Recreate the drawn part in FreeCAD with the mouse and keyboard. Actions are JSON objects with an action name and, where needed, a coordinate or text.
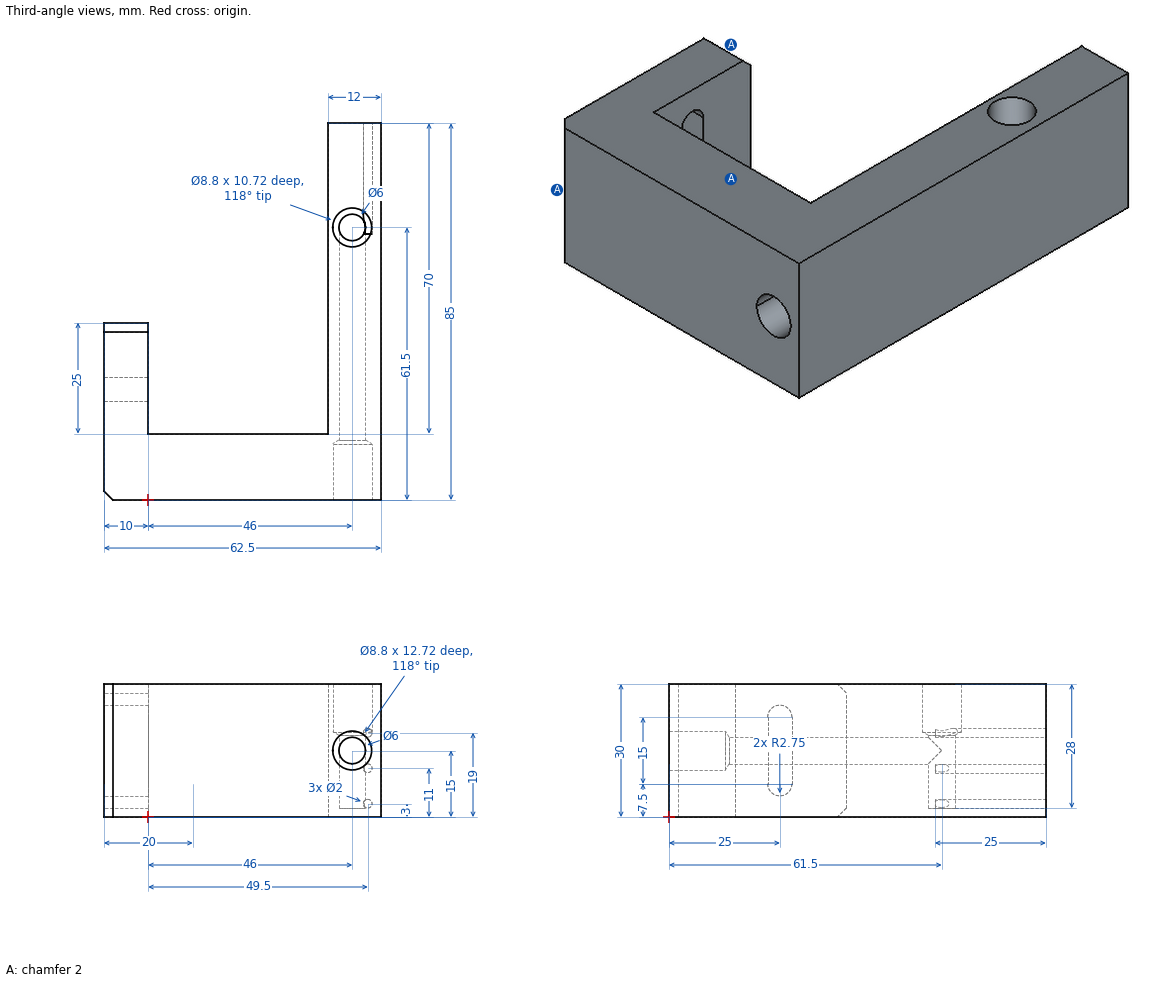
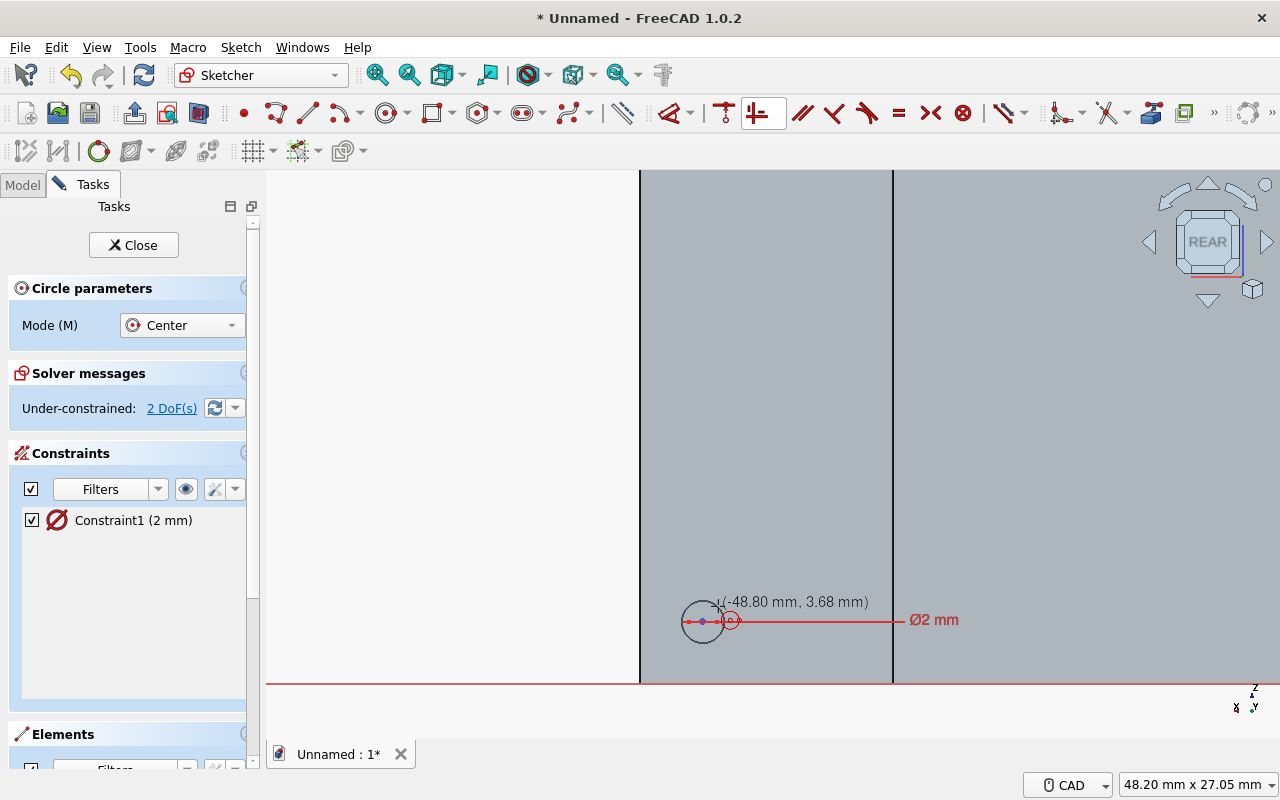
{"action": "left_click", "coordinate": [703, 453]}
{"action": "mouse_move", "coordinate": [718, 438]}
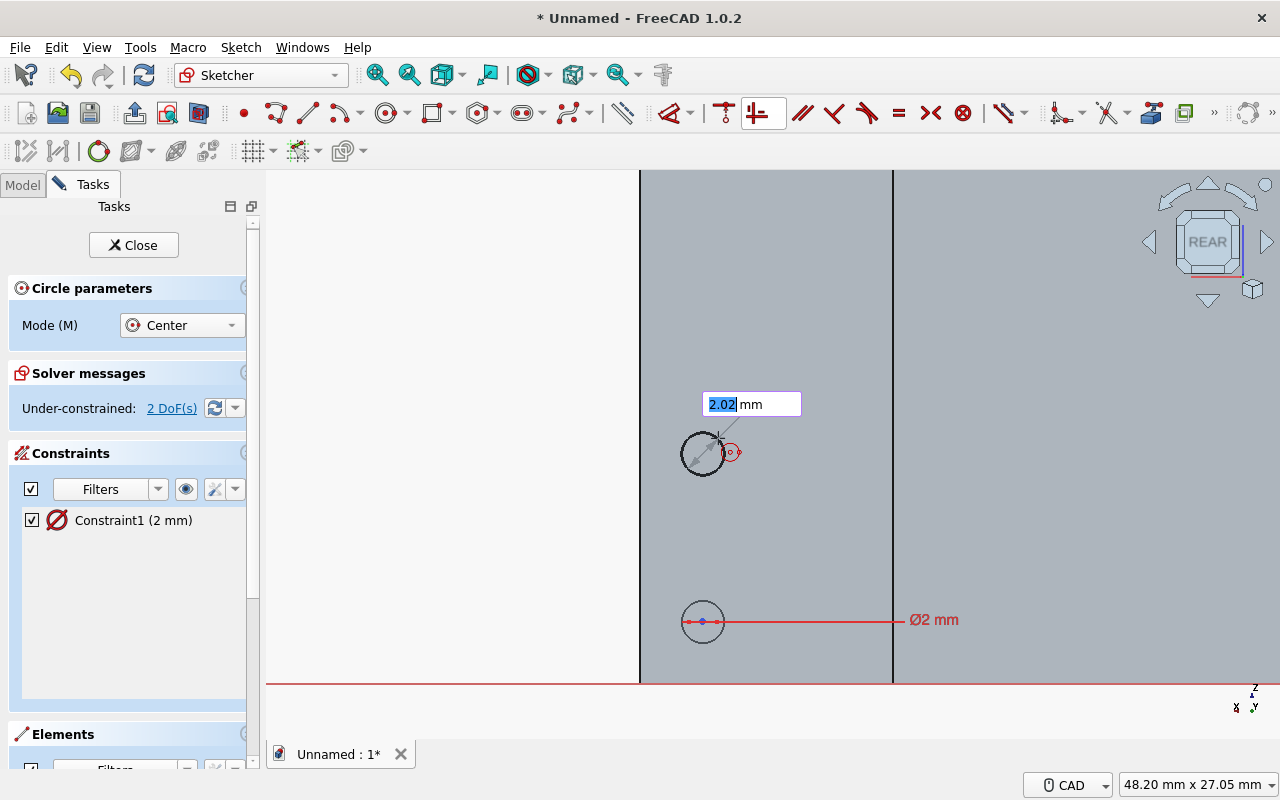
{"action": "type", "text": "2"}
{"action": "key", "text": "Return"}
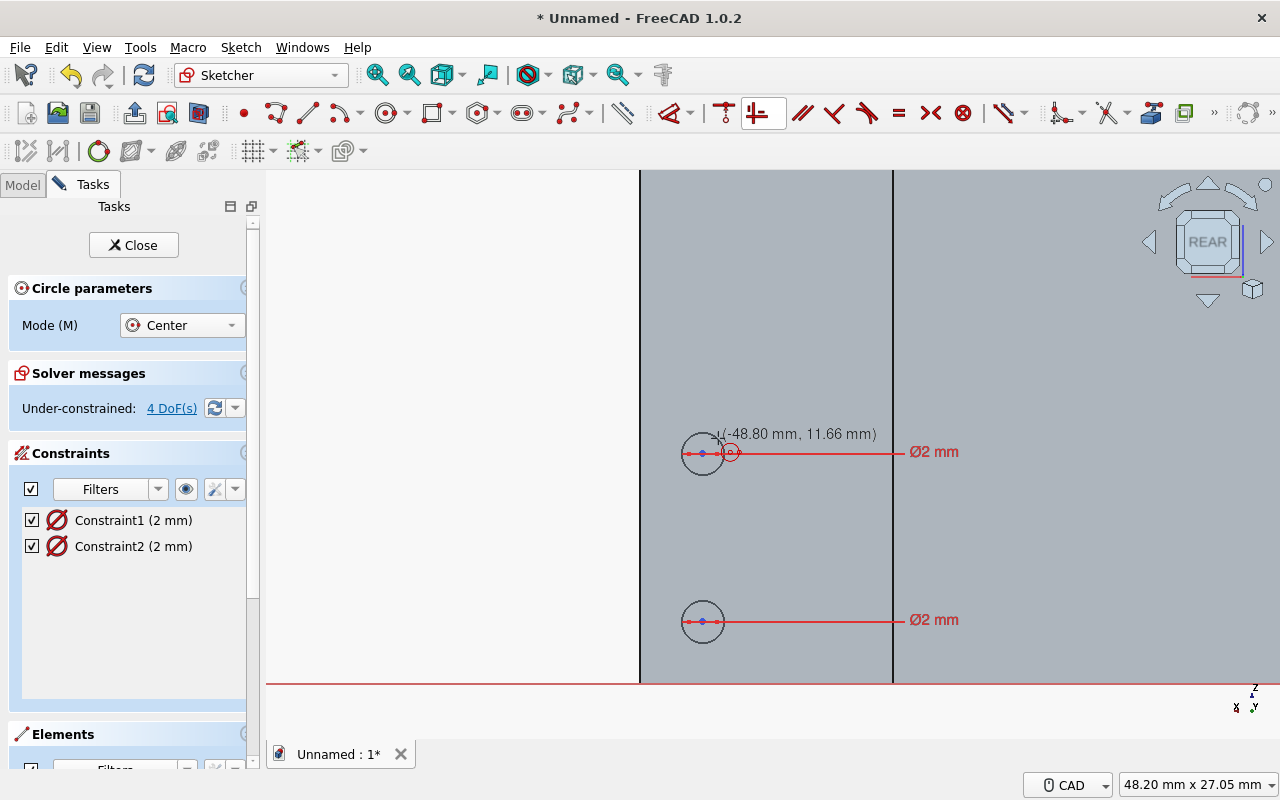
{"action": "left_click", "coordinate": [703, 285]}
{"action": "mouse_move", "coordinate": [718, 270]}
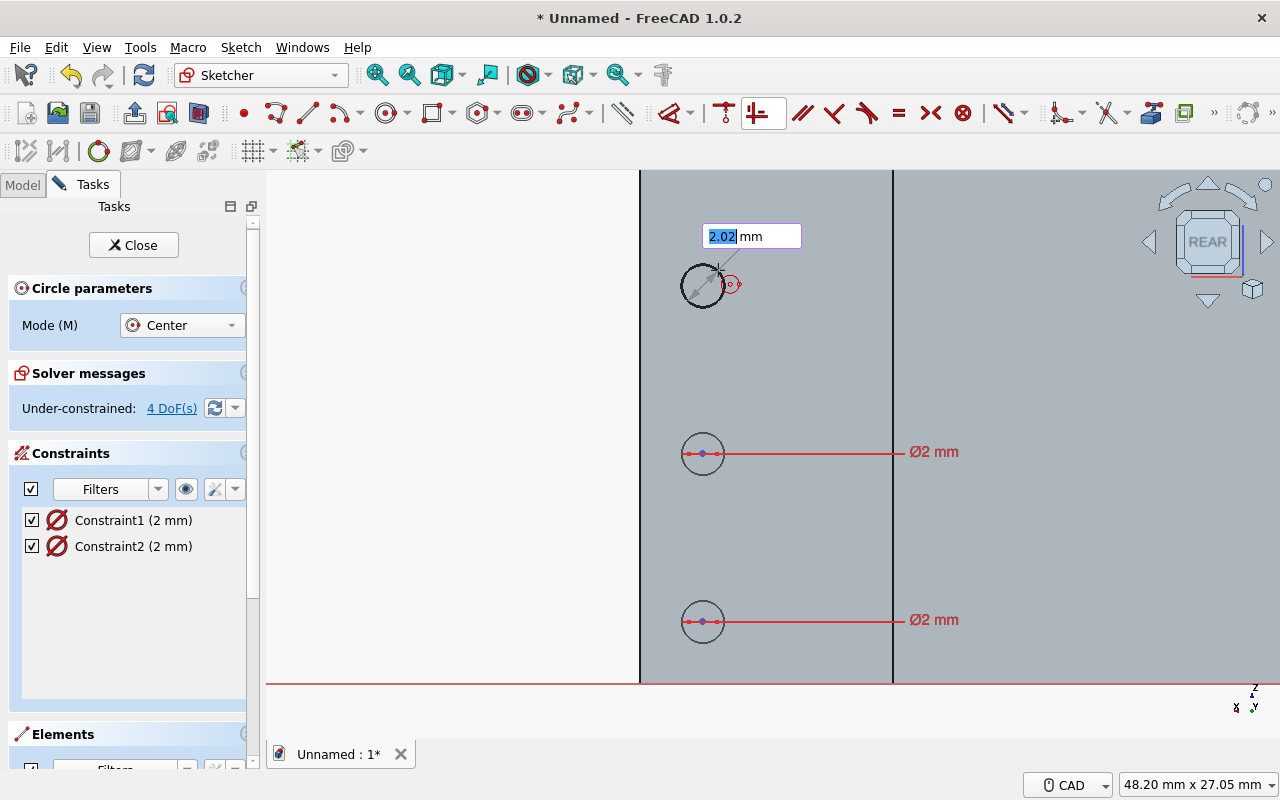
{"action": "type", "text": "2"}
{"action": "key", "text": "Return"}
{"action": "key", "text": "Escape"}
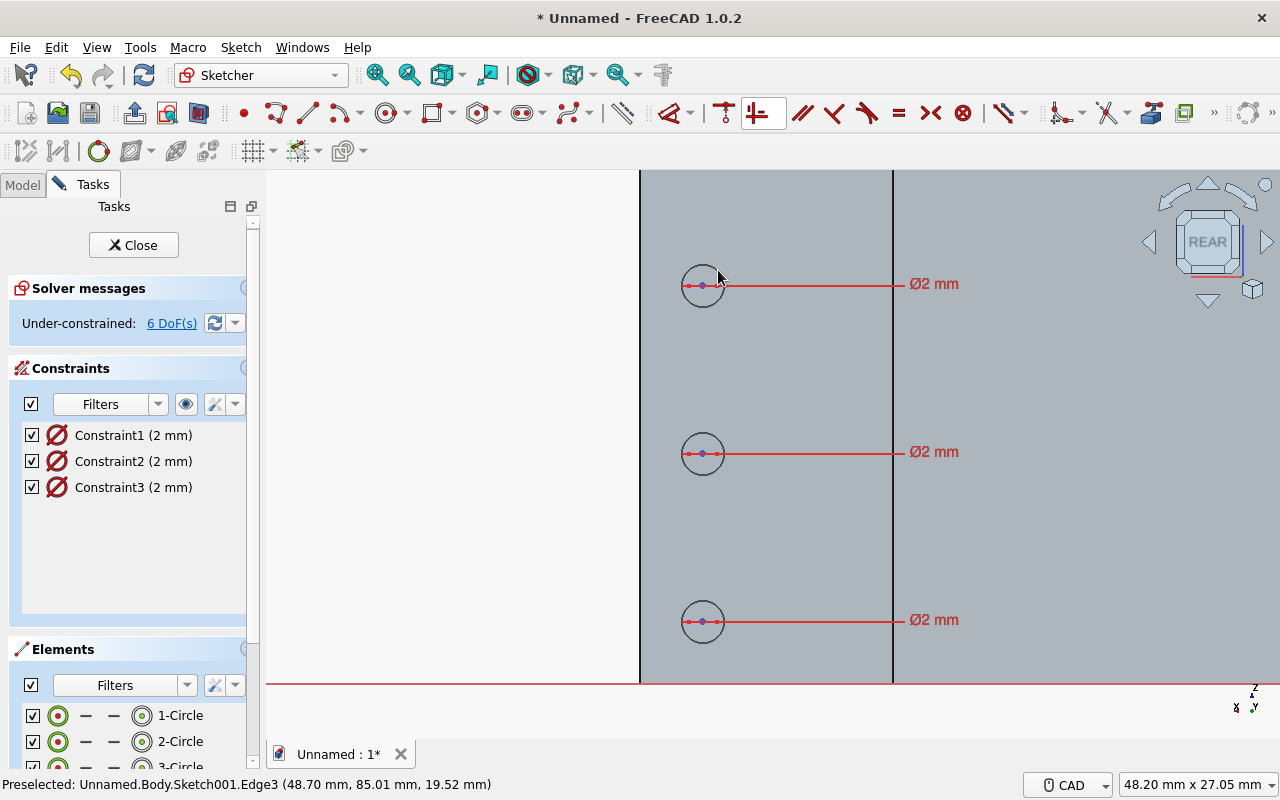
{"action": "key", "text": "d"}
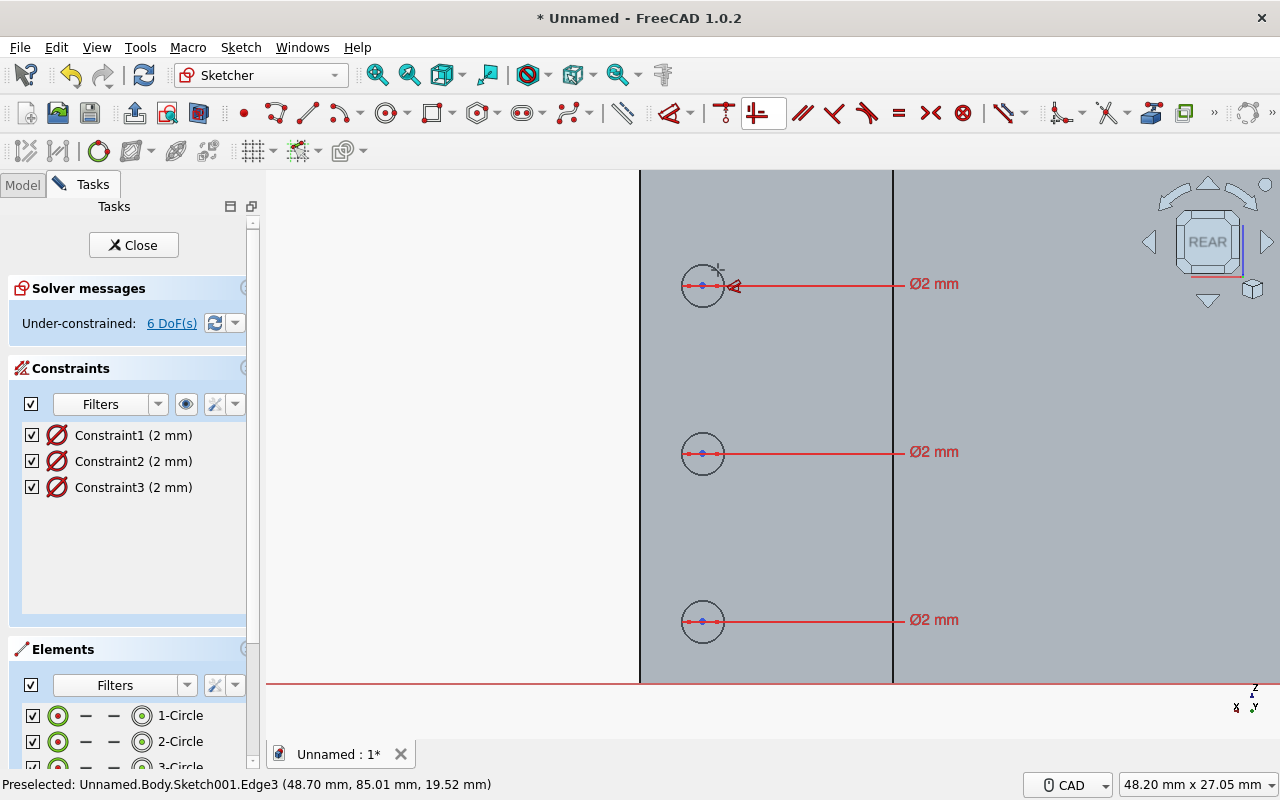
{"action": "left_click", "coordinate": [703, 622]}
{"action": "left_click", "coordinate": [669, 653]}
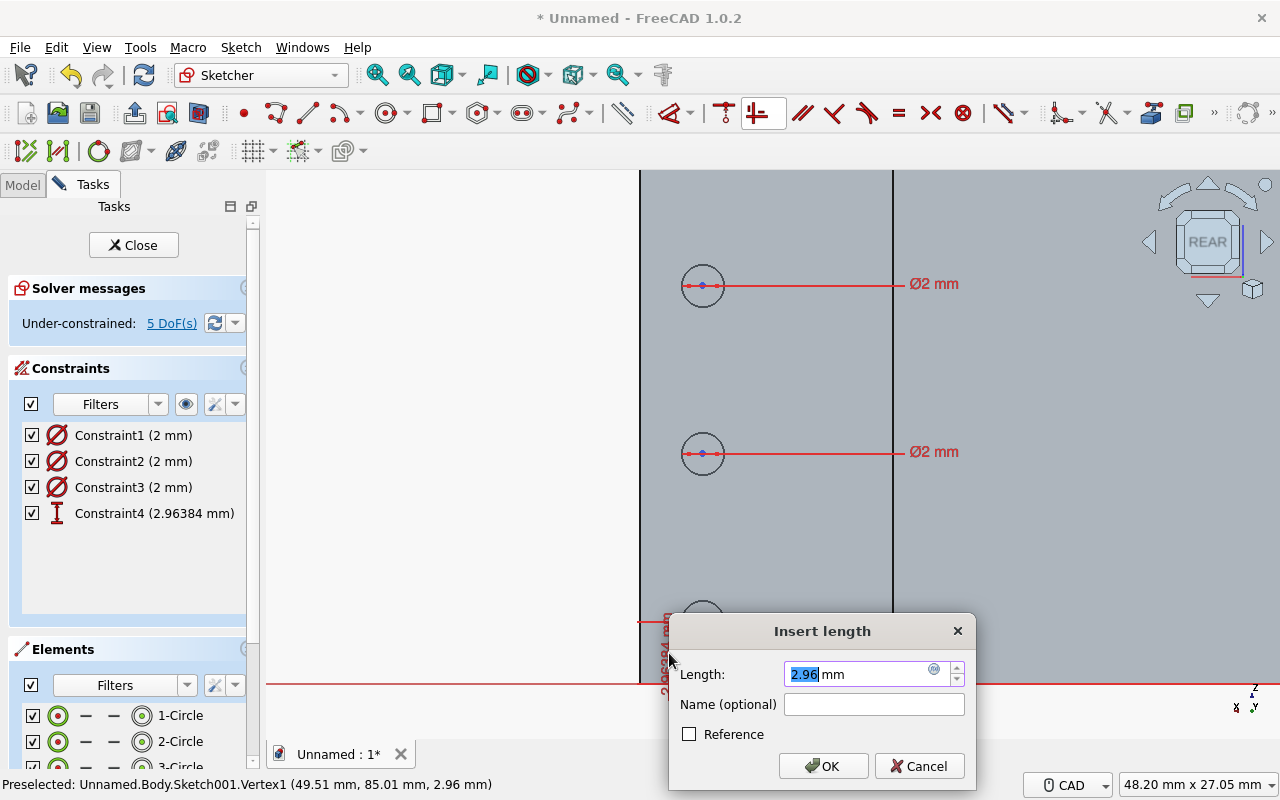
{"action": "type", "text": "3"}
{"action": "key", "text": "Return"}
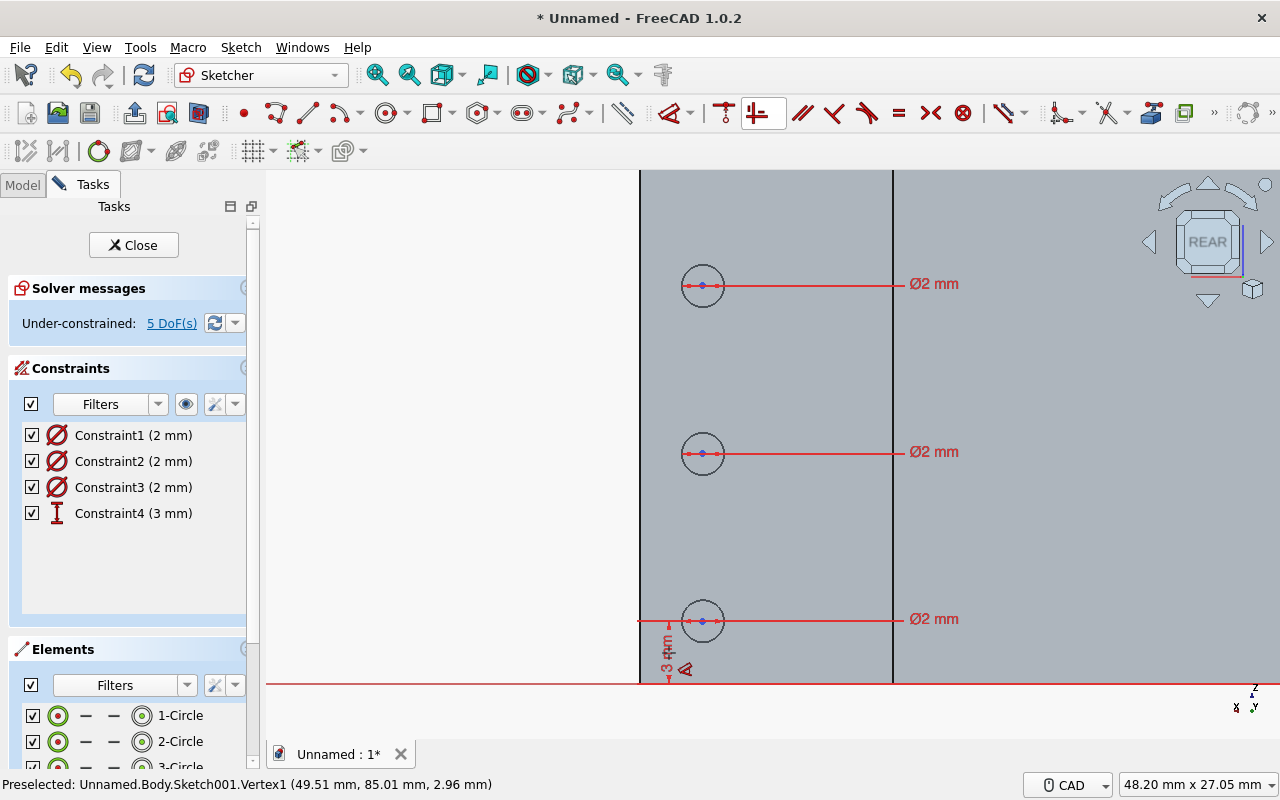
{"action": "left_click", "coordinate": [703, 454]}
{"action": "left_click", "coordinate": [669, 569]}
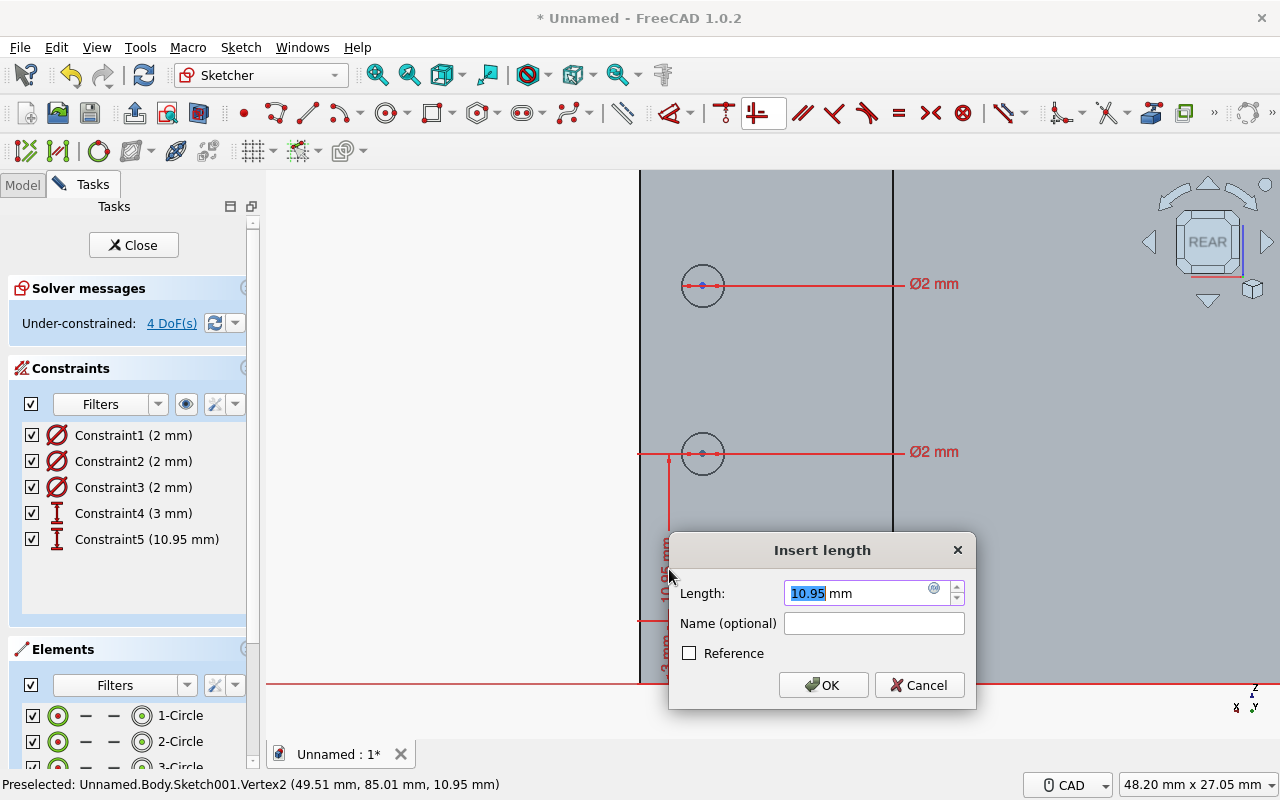
{"action": "type", "text": "11"}
{"action": "key", "text": "Return"}